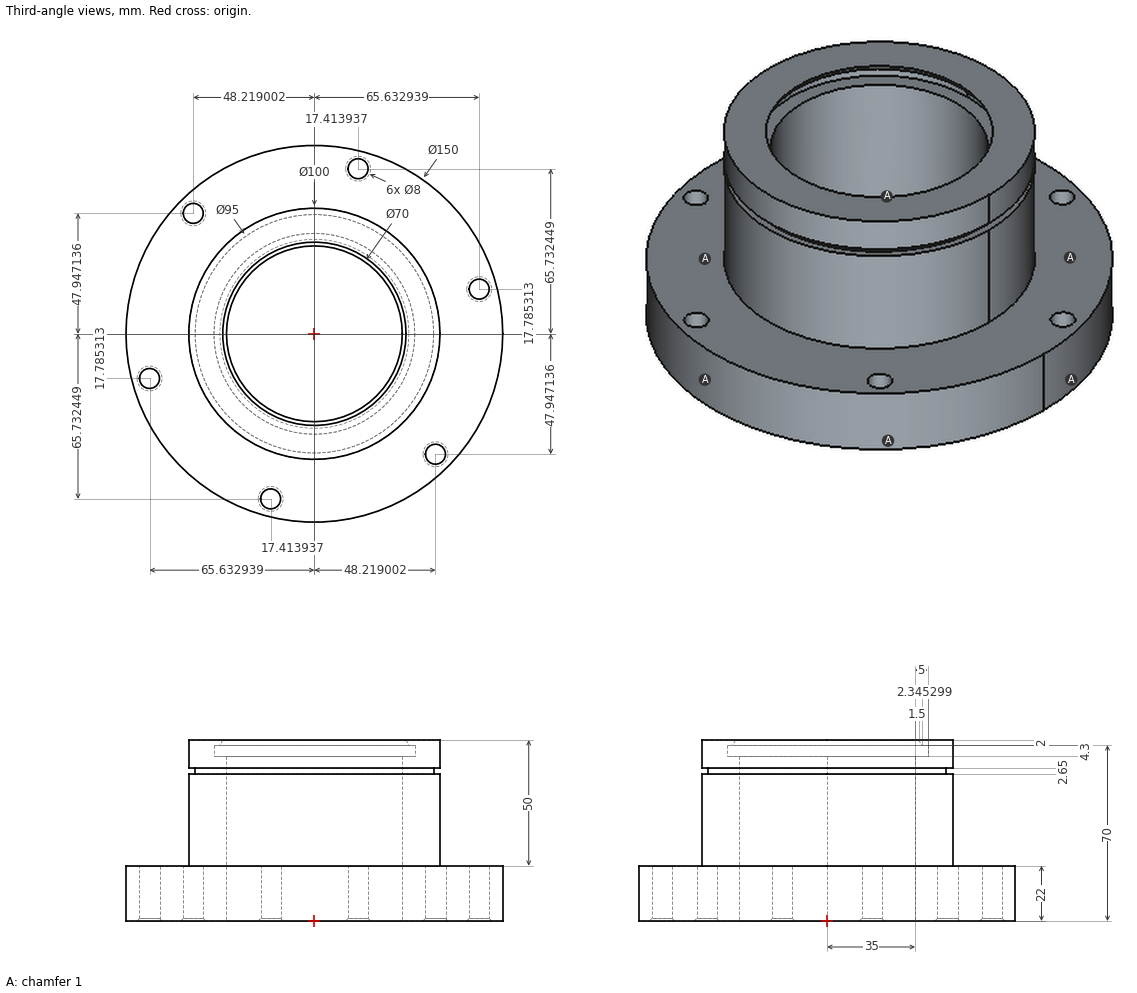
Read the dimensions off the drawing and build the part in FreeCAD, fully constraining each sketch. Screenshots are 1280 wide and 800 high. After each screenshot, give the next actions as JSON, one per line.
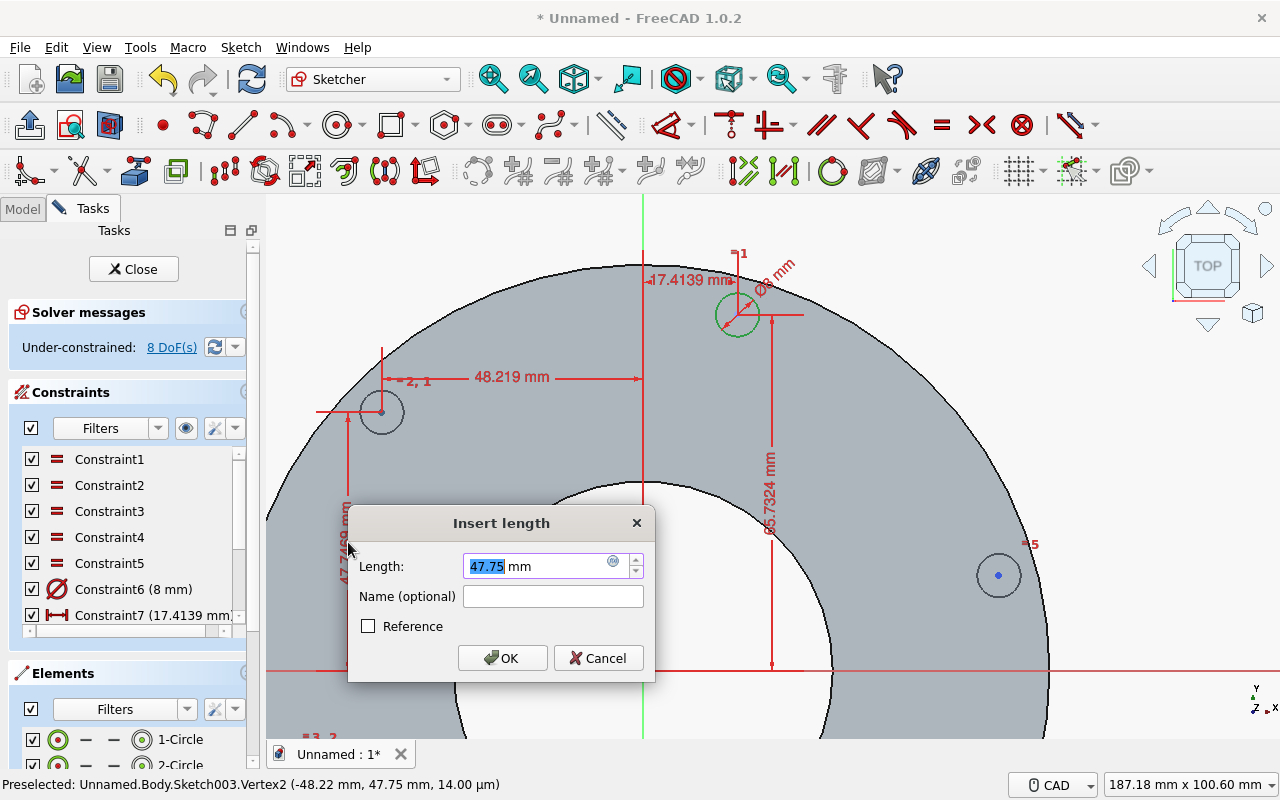
{"action": "type", "text": "47.947136"}
{"action": "key", "text": "Return"}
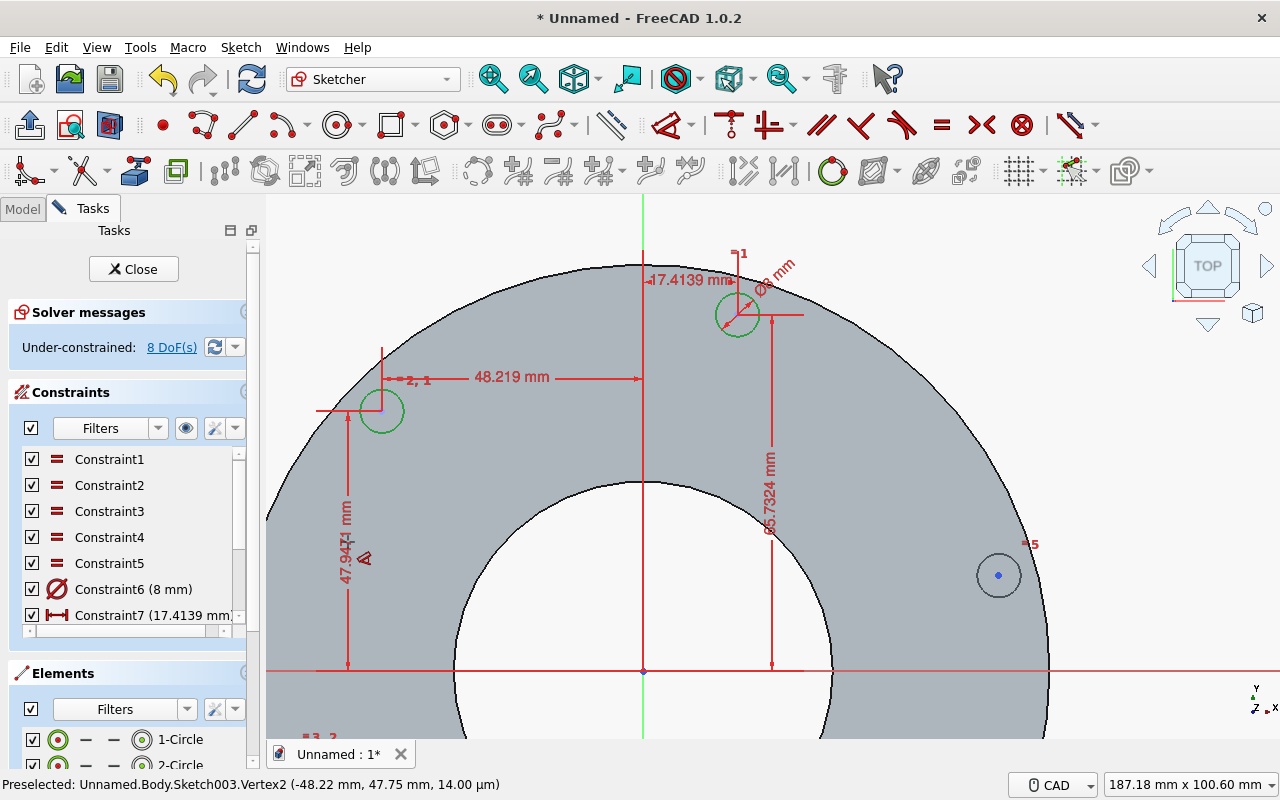
{"action": "scroll", "coordinate": [755, 300], "scroll_direction": "down", "scroll_amount": 4}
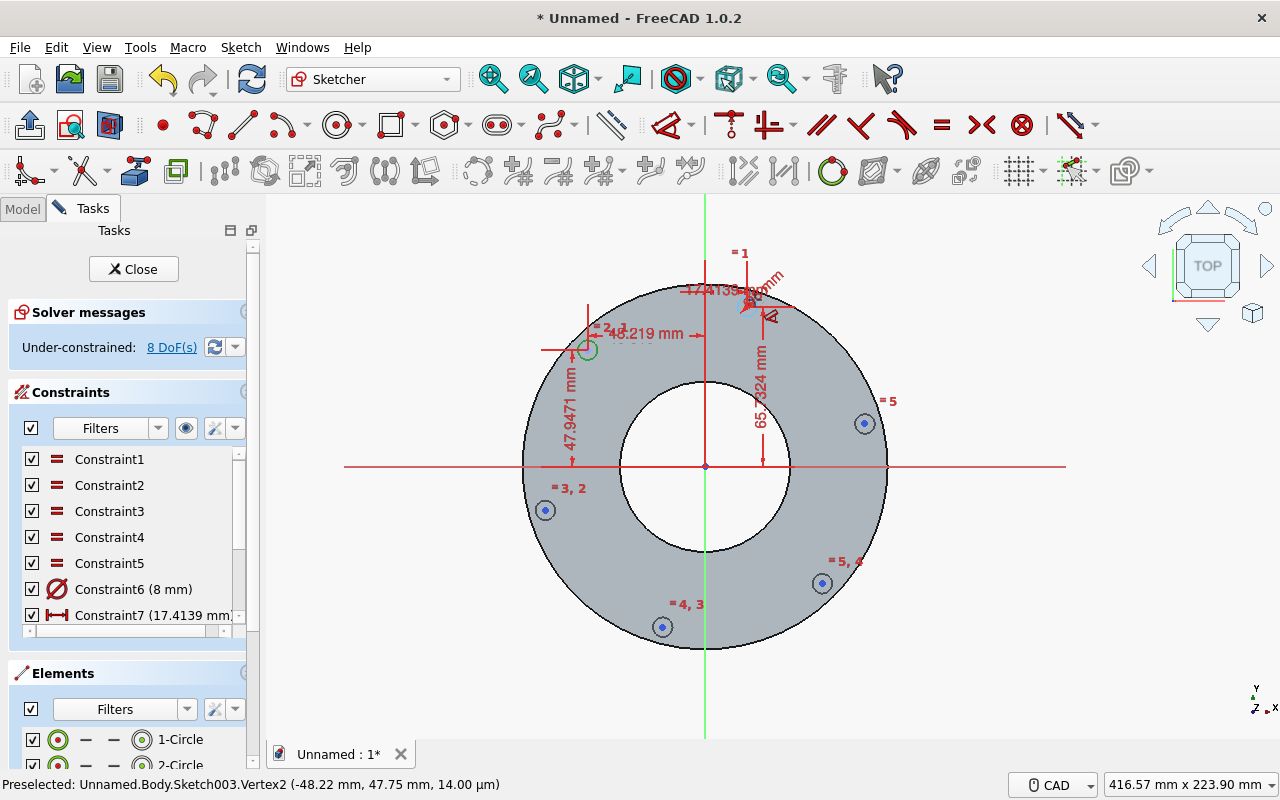
{"action": "left_click", "coordinate": [545, 510]}
{"action": "left_click", "coordinate": [625, 544]}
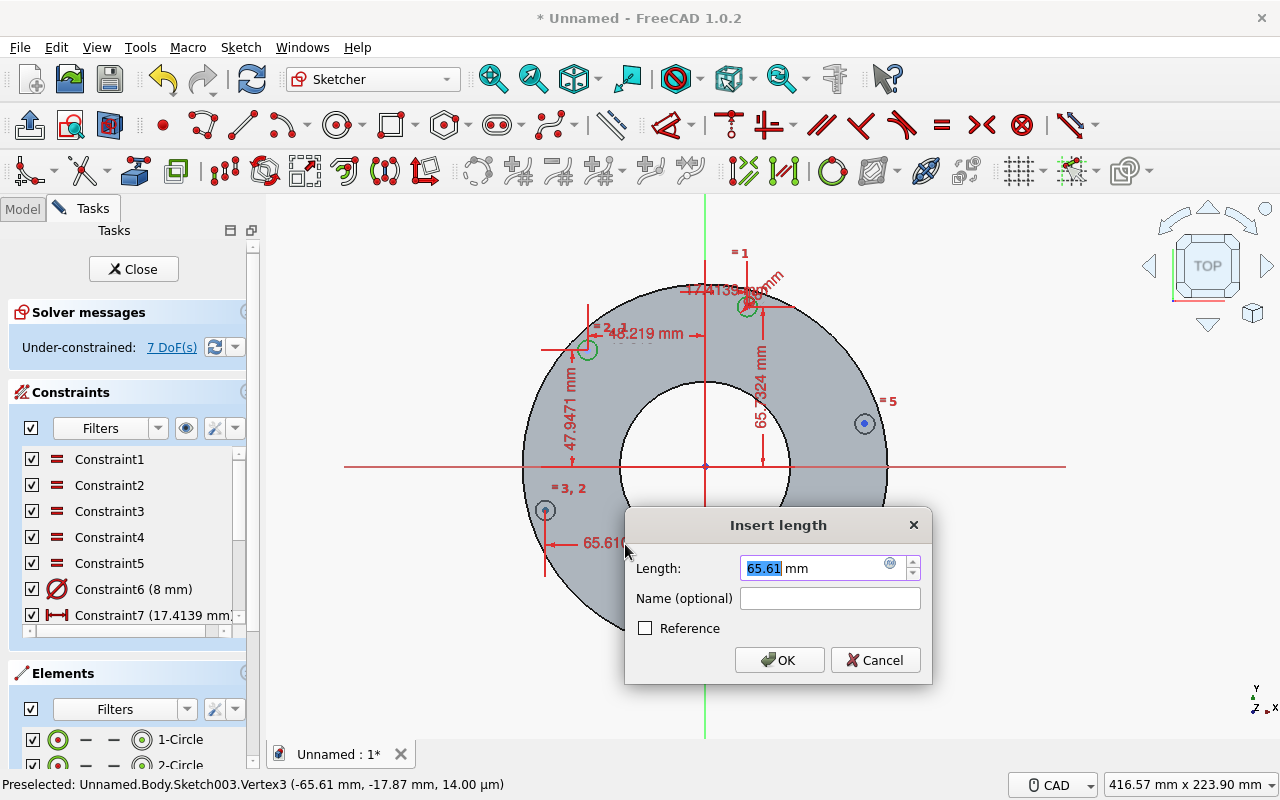
{"action": "type", "text": "65.632939"}
{"action": "key", "text": "Return"}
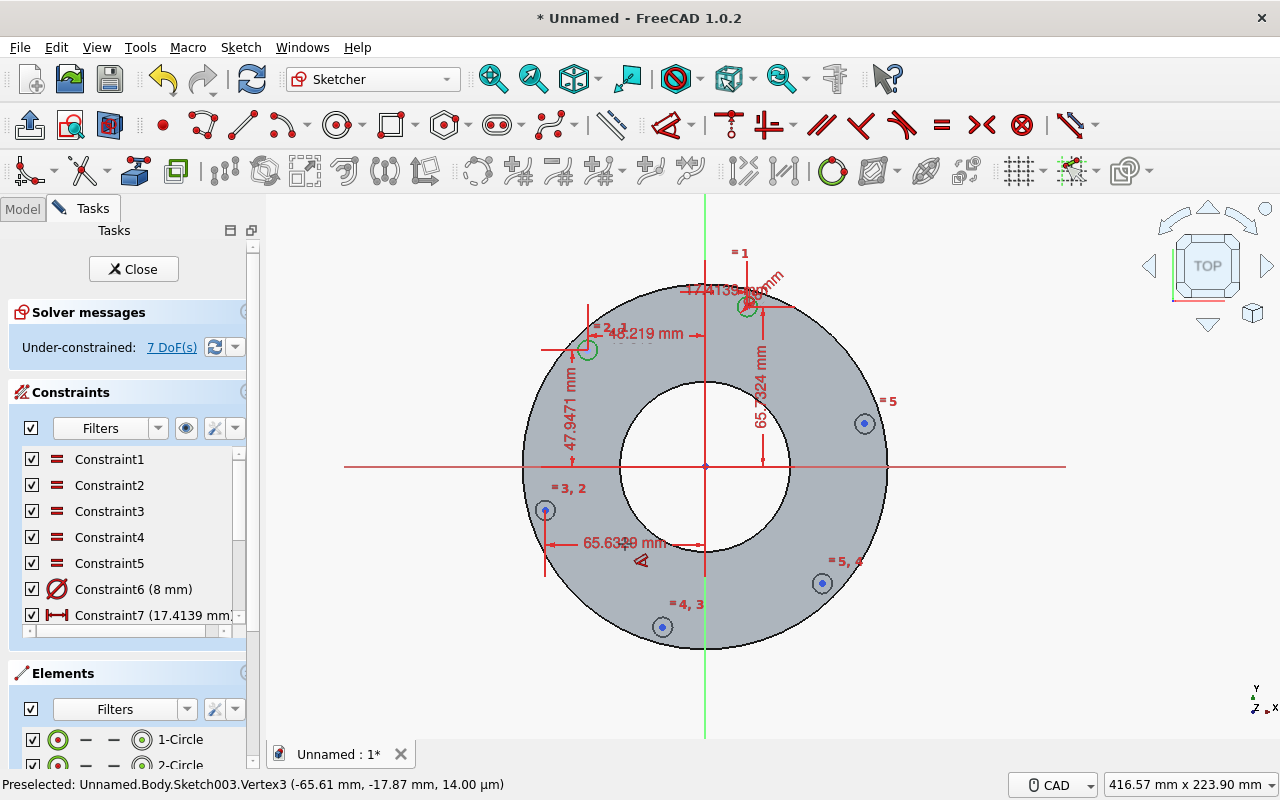
{"action": "left_click", "coordinate": [545, 510]}
{"action": "left_click", "coordinate": [511, 489]}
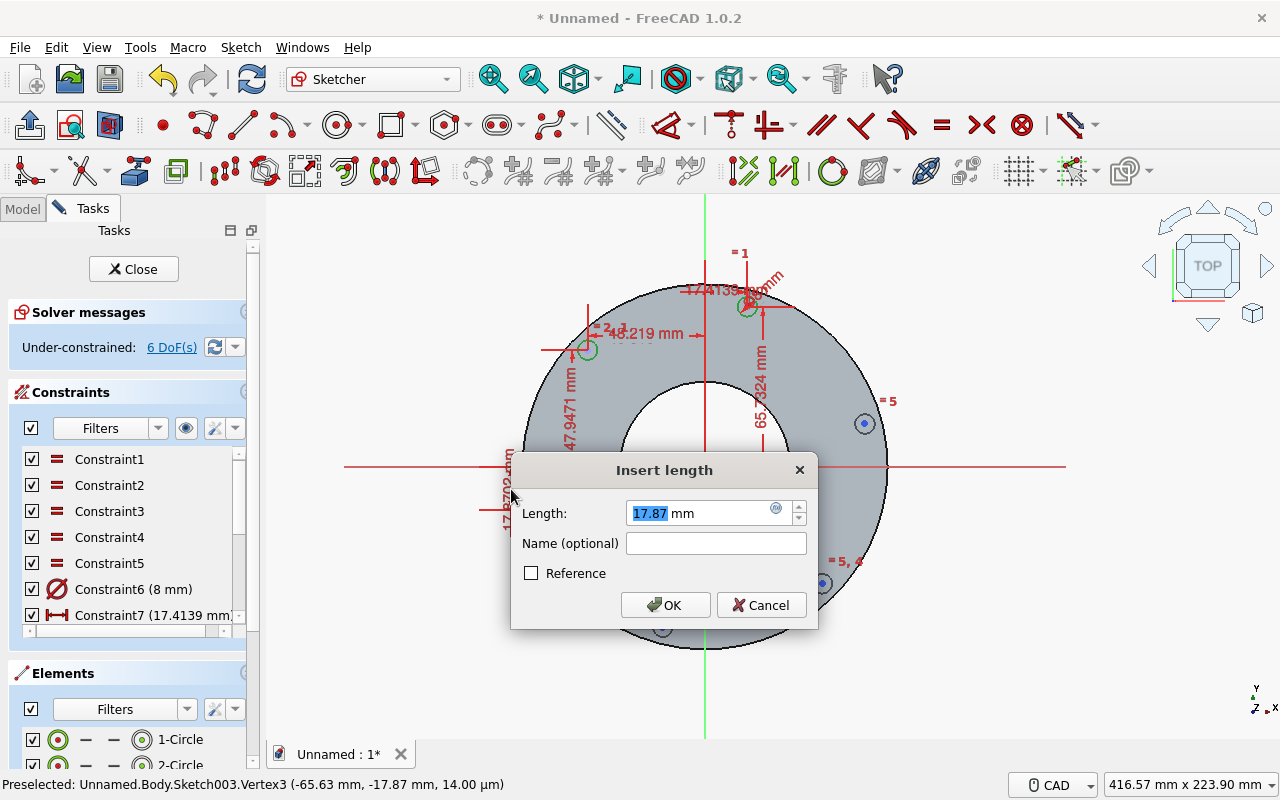
{"action": "type", "text": "17.785313"}
{"action": "key", "text": "Return"}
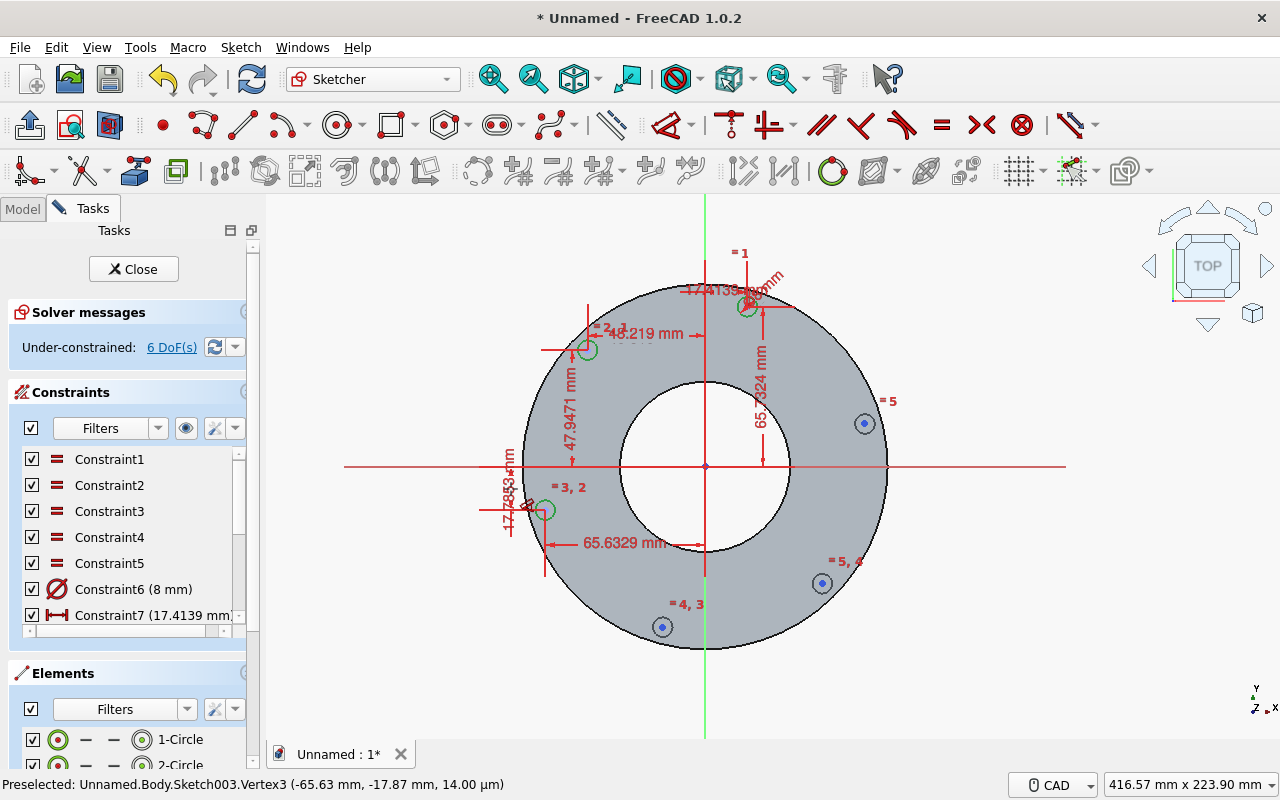
{"action": "left_click", "coordinate": [663, 627]}
{"action": "left_click", "coordinate": [684, 661]}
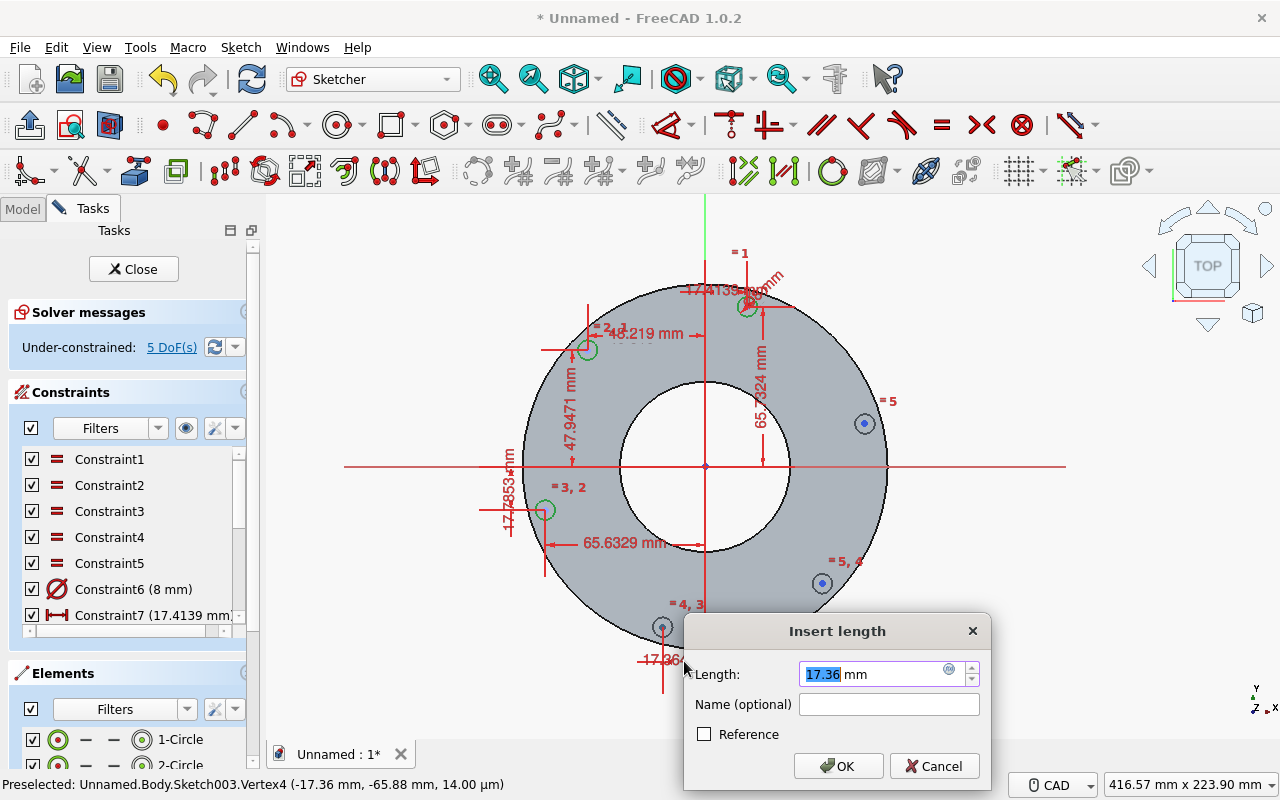
{"action": "type", "text": "17.413937"}
{"action": "key", "text": "Return"}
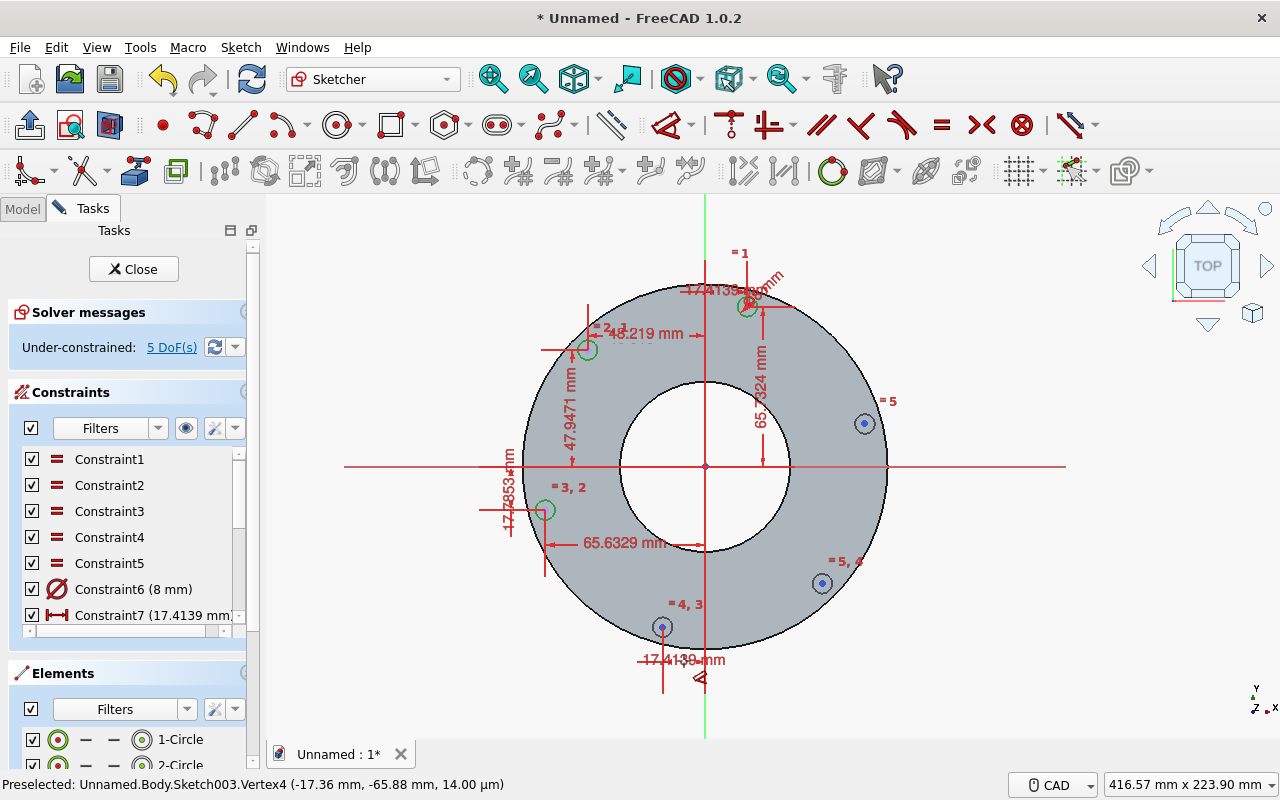
{"action": "left_click", "coordinate": [663, 627]}
{"action": "left_click", "coordinate": [629, 510]}